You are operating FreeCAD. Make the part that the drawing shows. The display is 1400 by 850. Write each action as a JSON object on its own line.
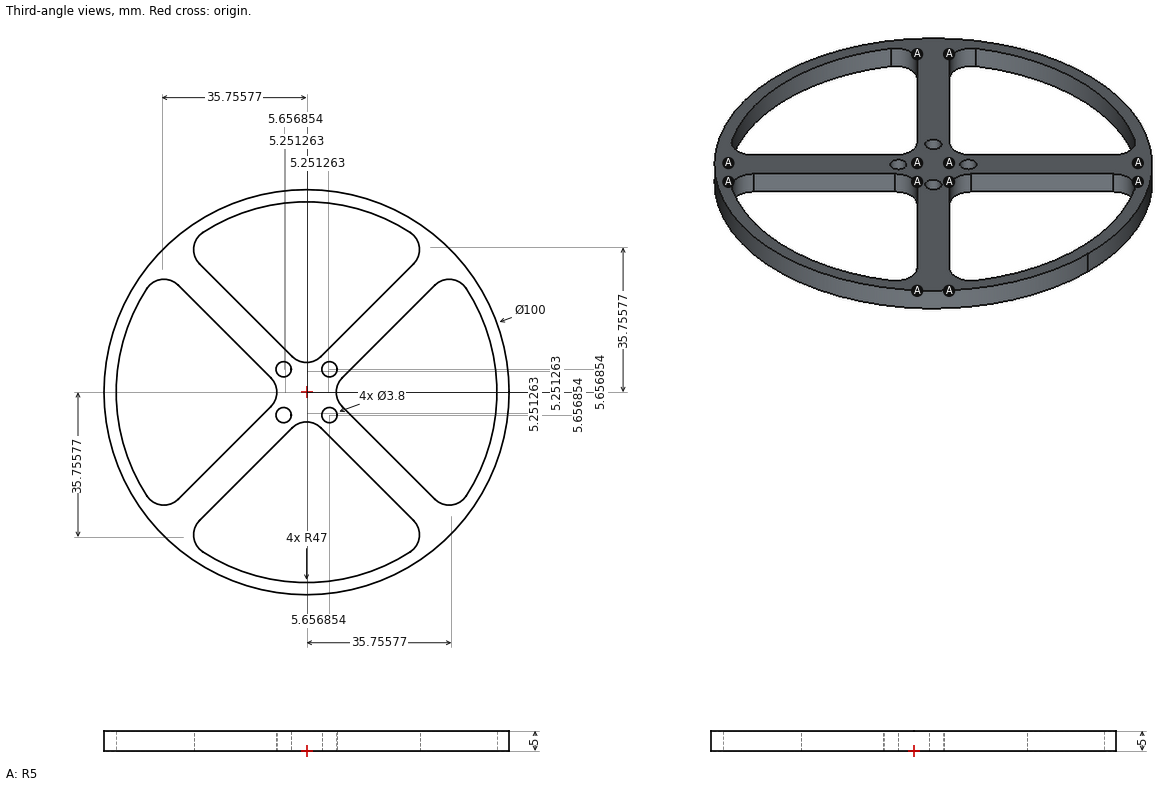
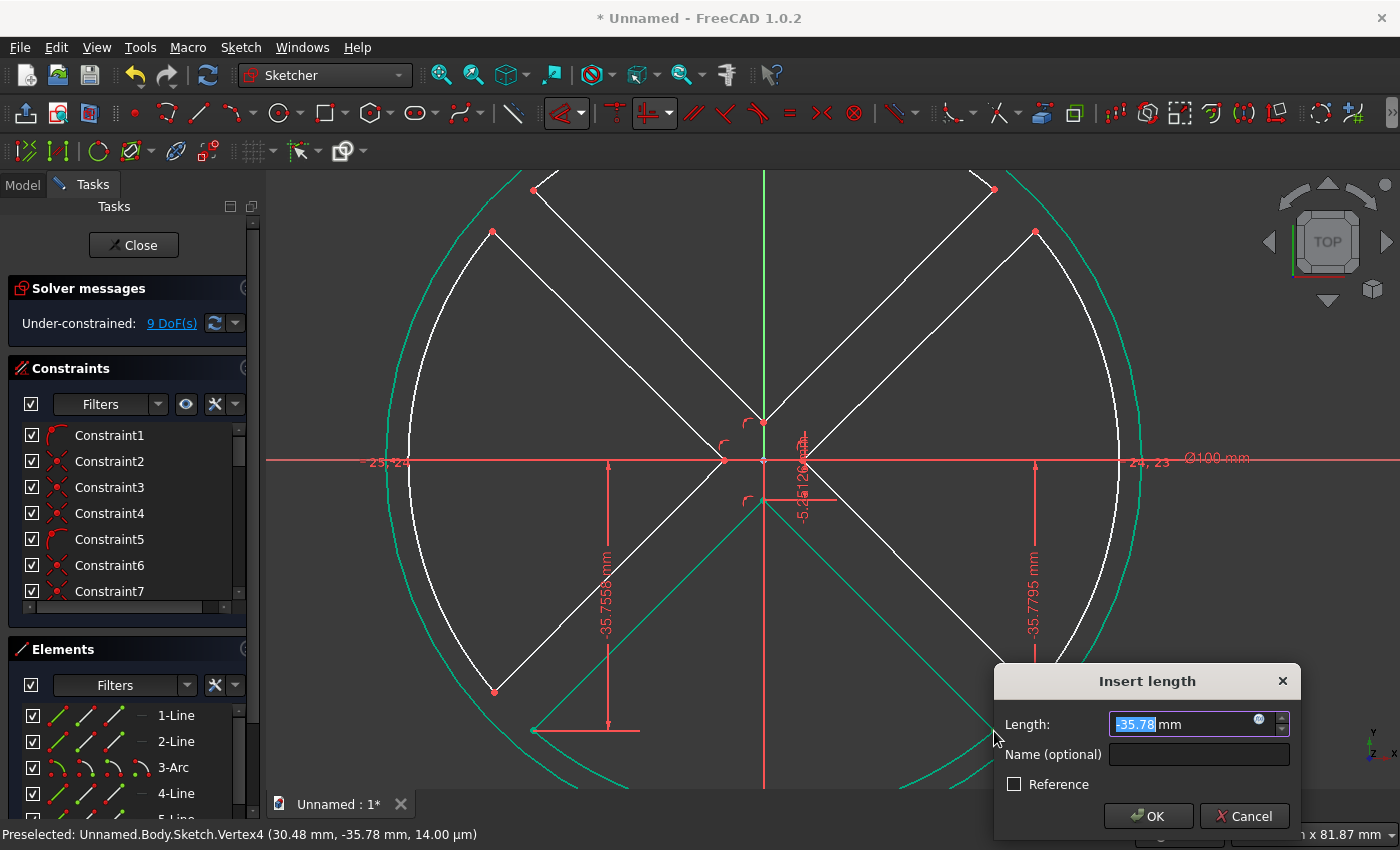
{"action": "type", "text": "-35.75577"}
{"action": "key", "text": "Return"}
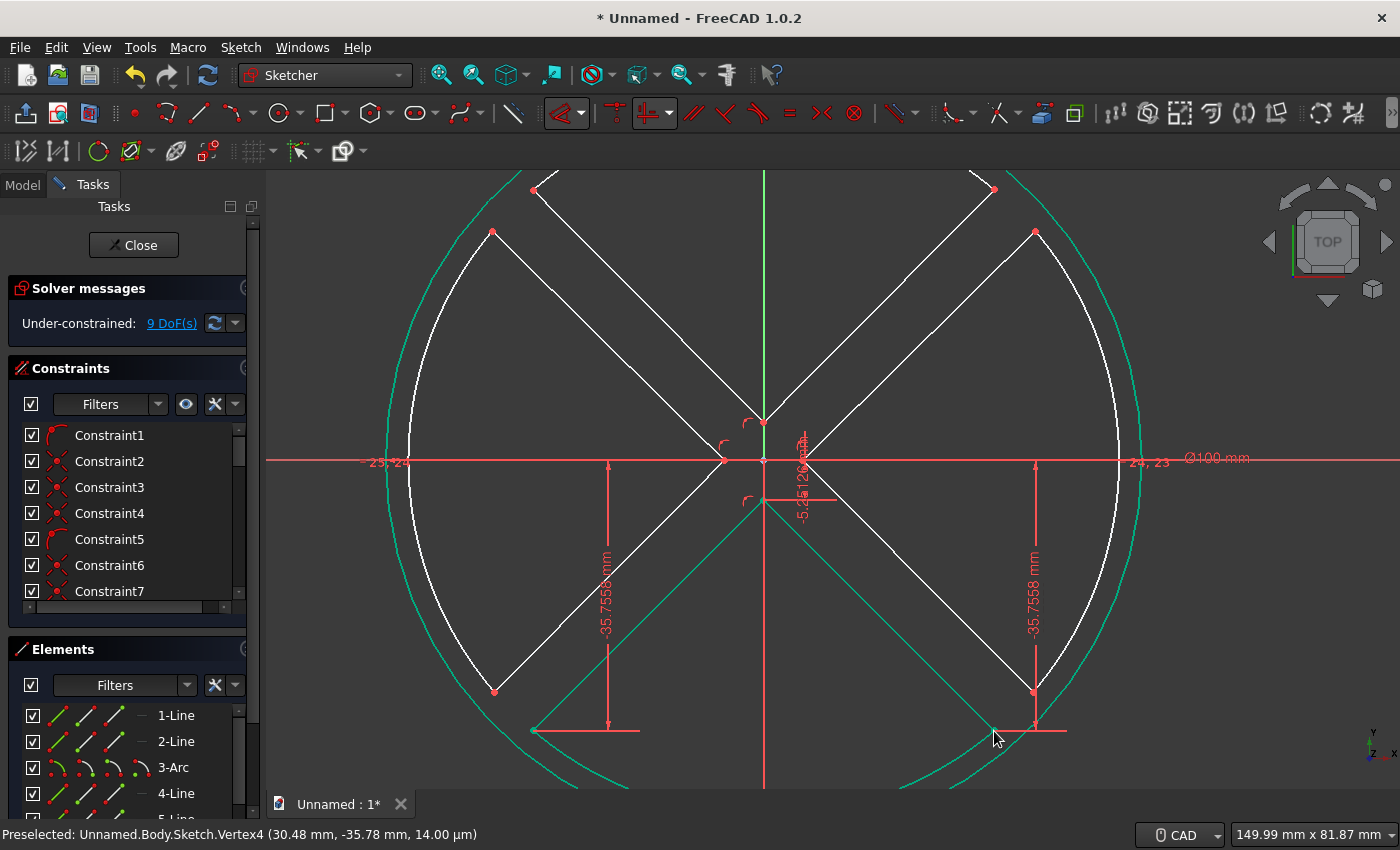
{"action": "left_click", "coordinate": [1033, 692]}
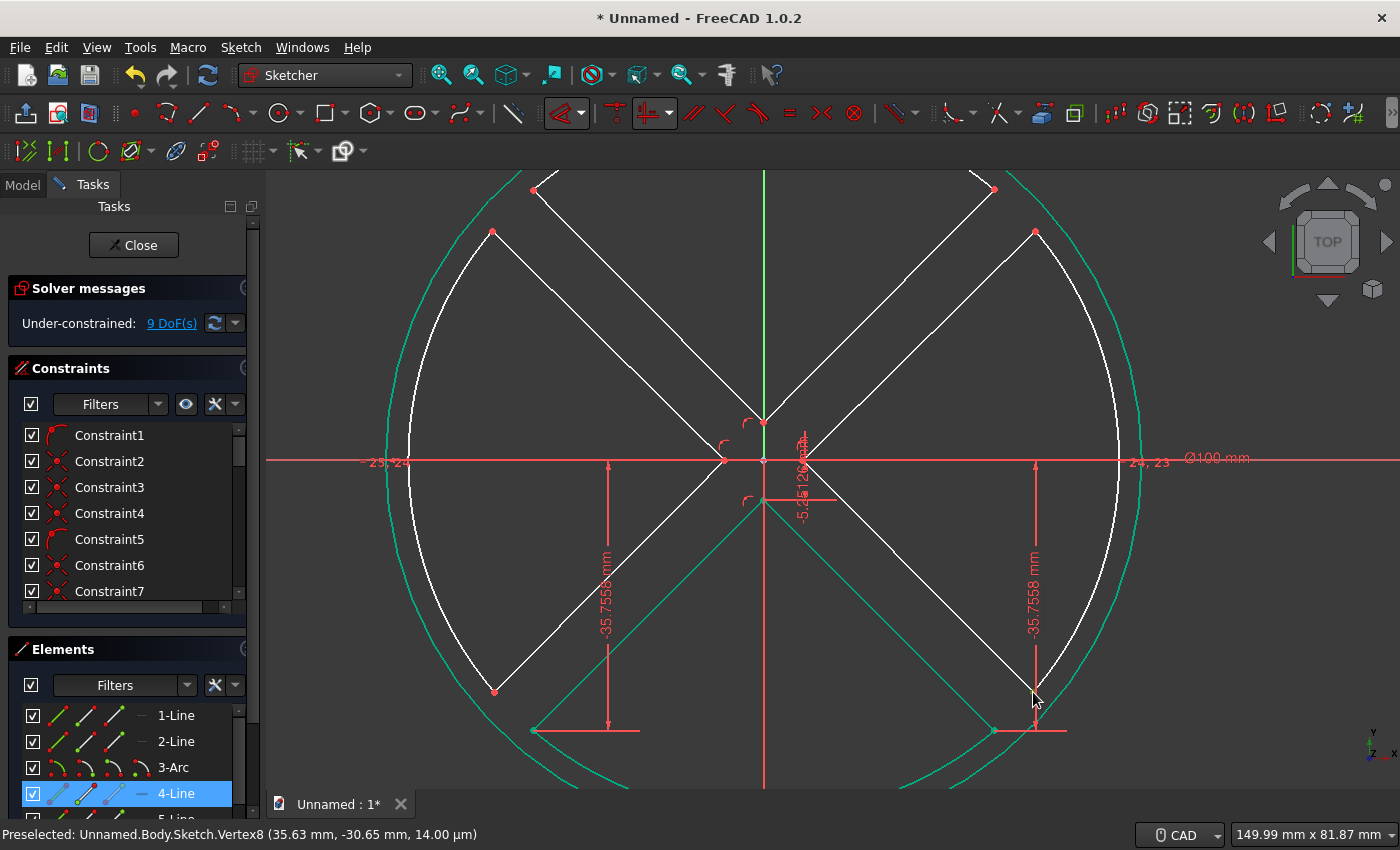
{"action": "key", "text": "l"}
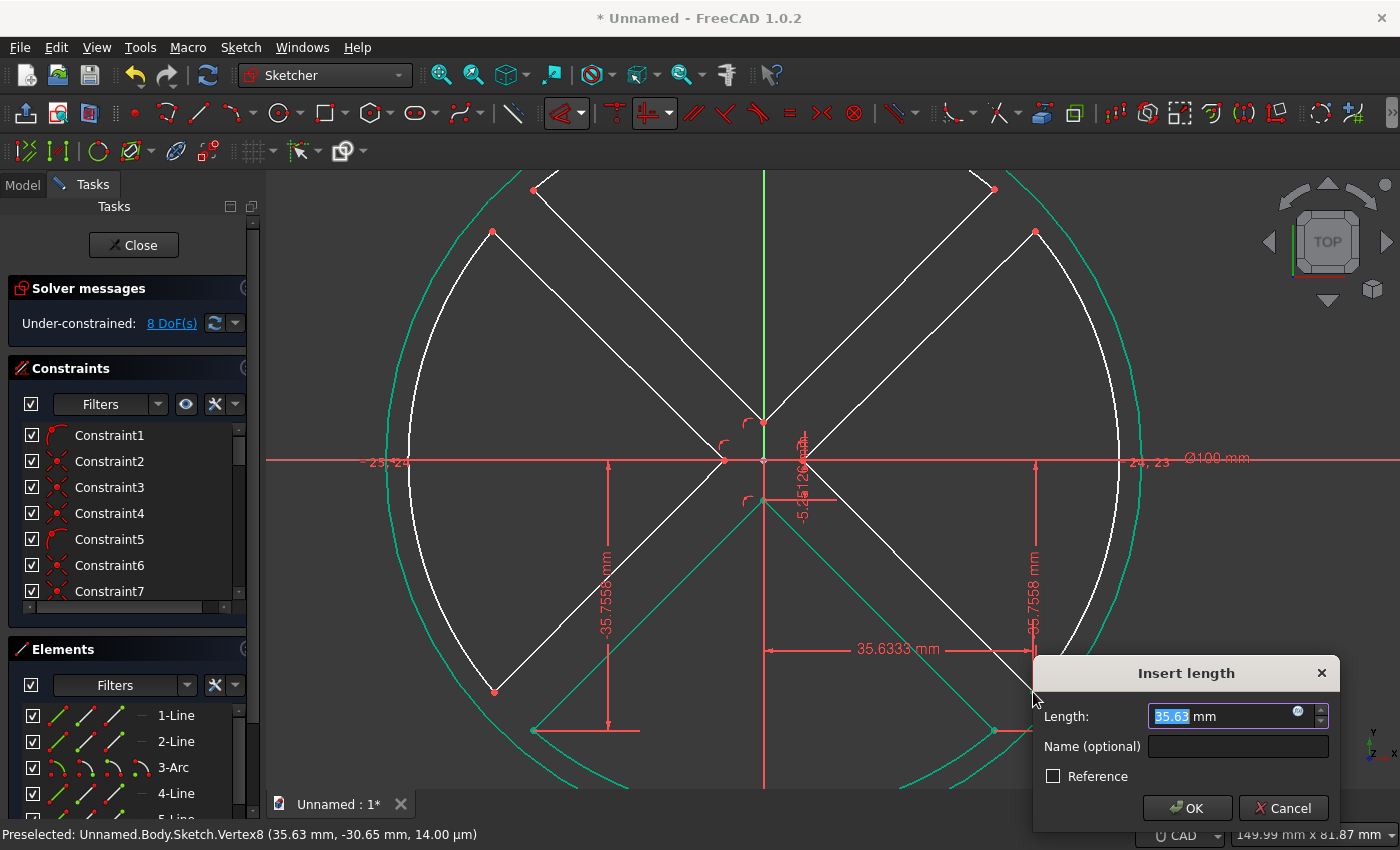
{"action": "type", "text": "35.75577"}
{"action": "key", "text": "Return"}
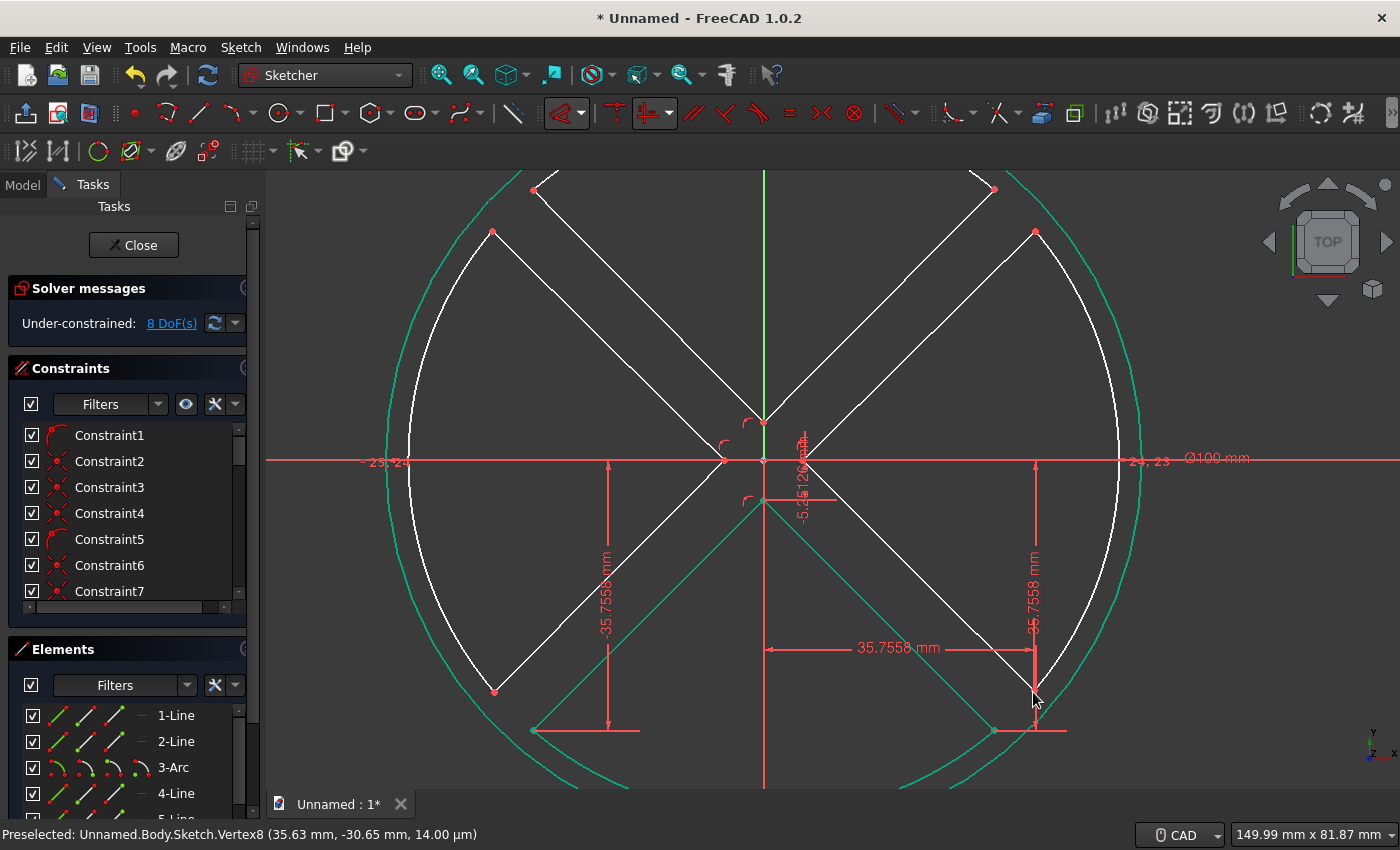
{"action": "left_click", "coordinate": [803, 460]}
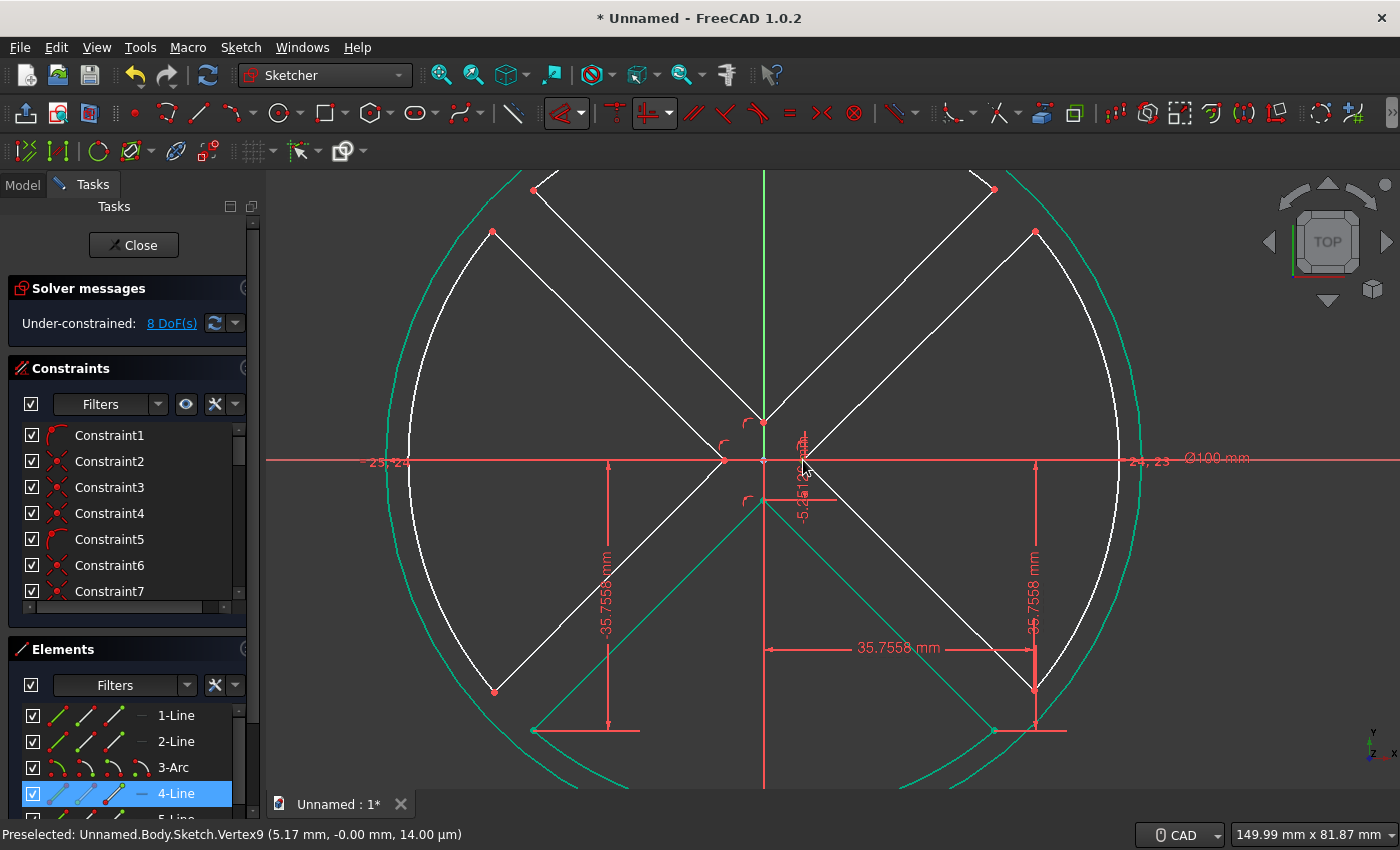
{"action": "key", "text": "l"}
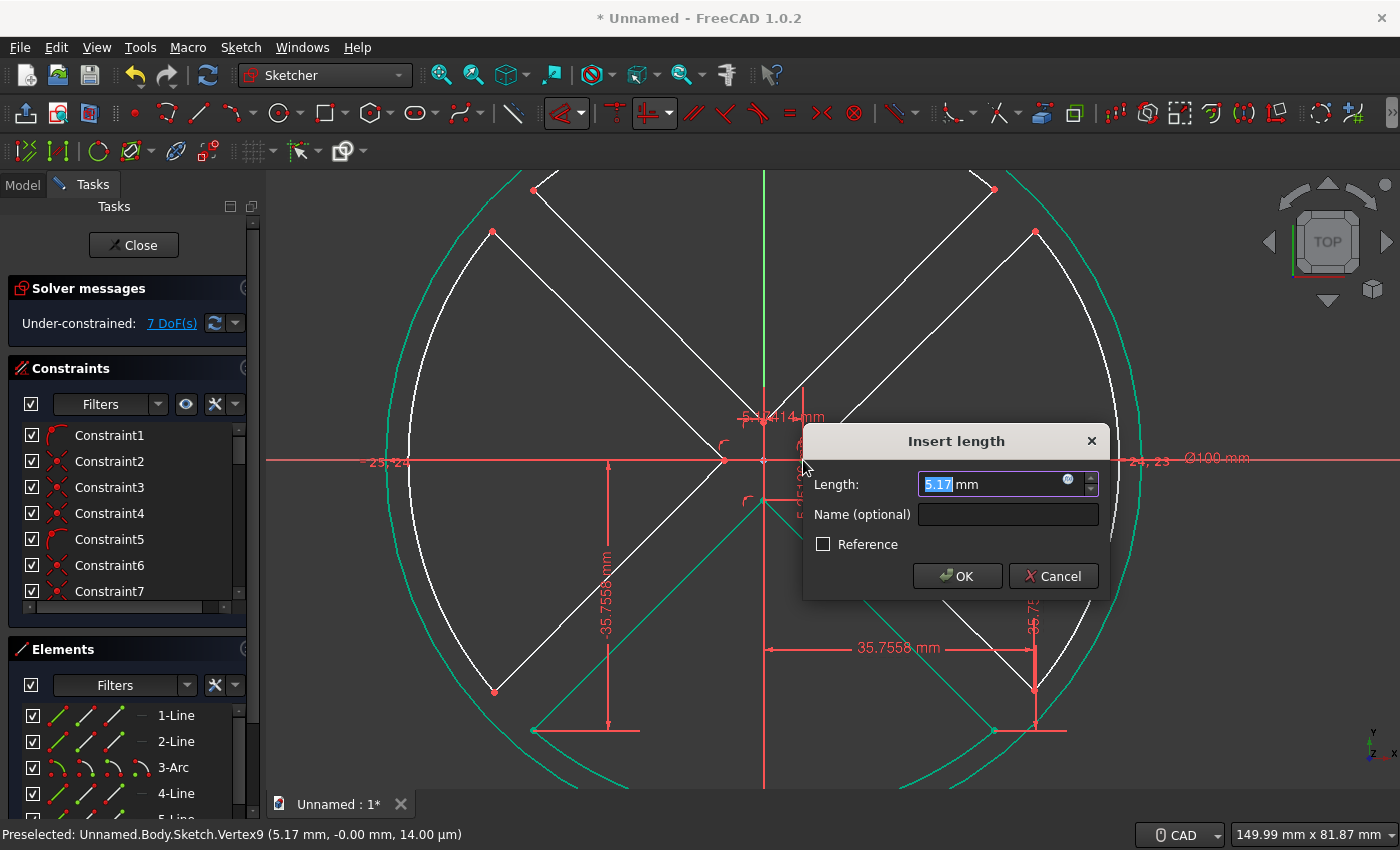
{"action": "type", "text": "5.251263"}
{"action": "key", "text": "Return"}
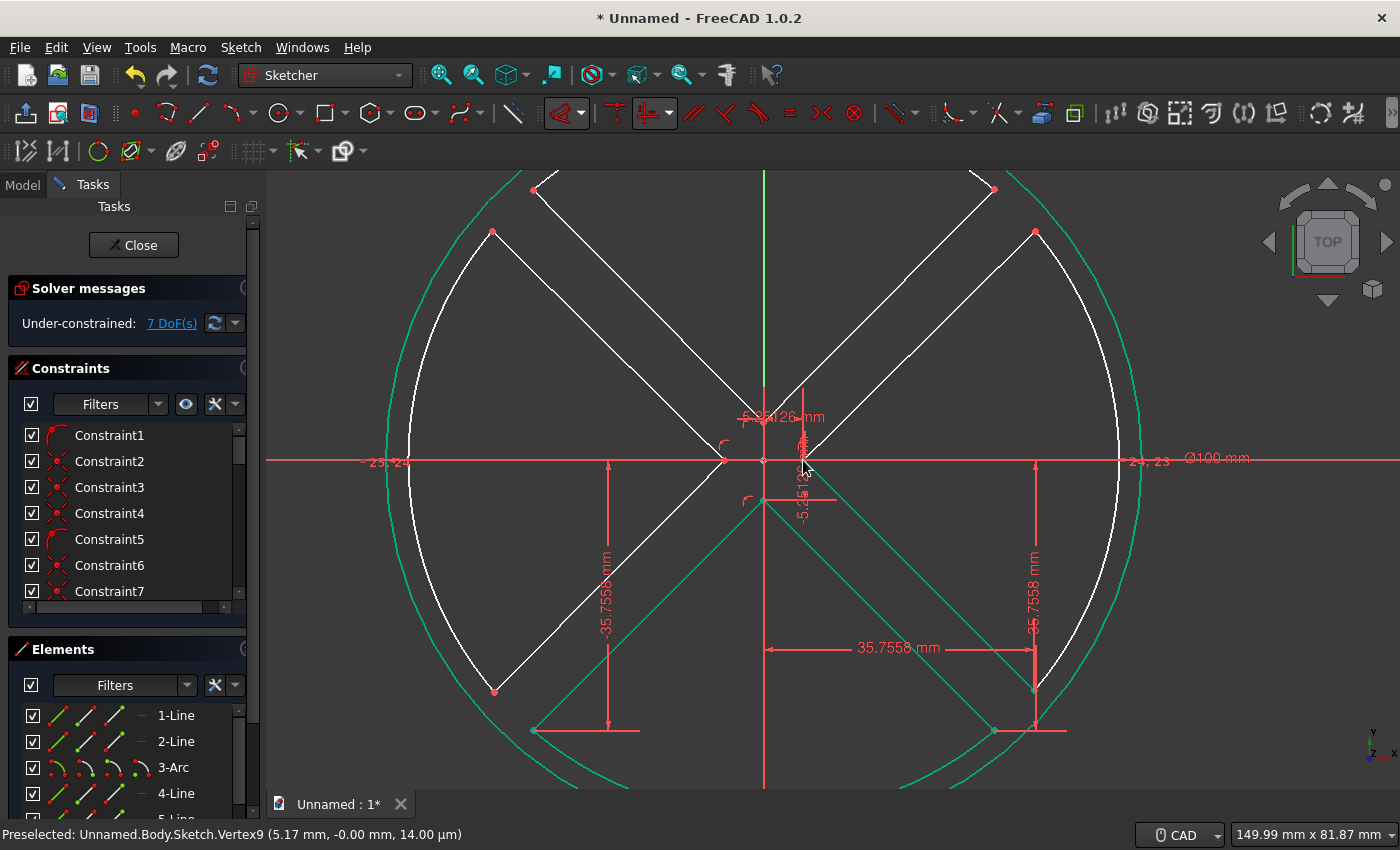
{"action": "left_click", "coordinate": [1035, 231]}